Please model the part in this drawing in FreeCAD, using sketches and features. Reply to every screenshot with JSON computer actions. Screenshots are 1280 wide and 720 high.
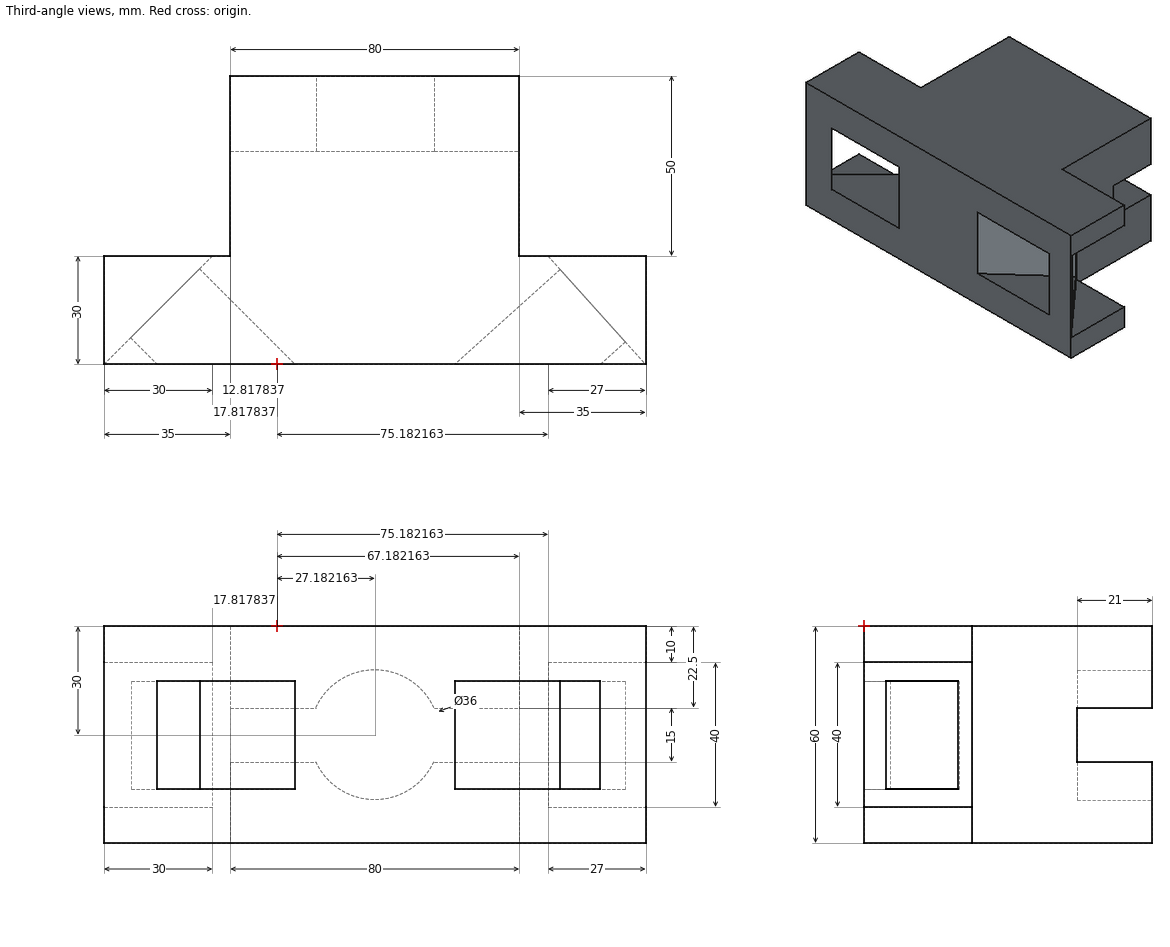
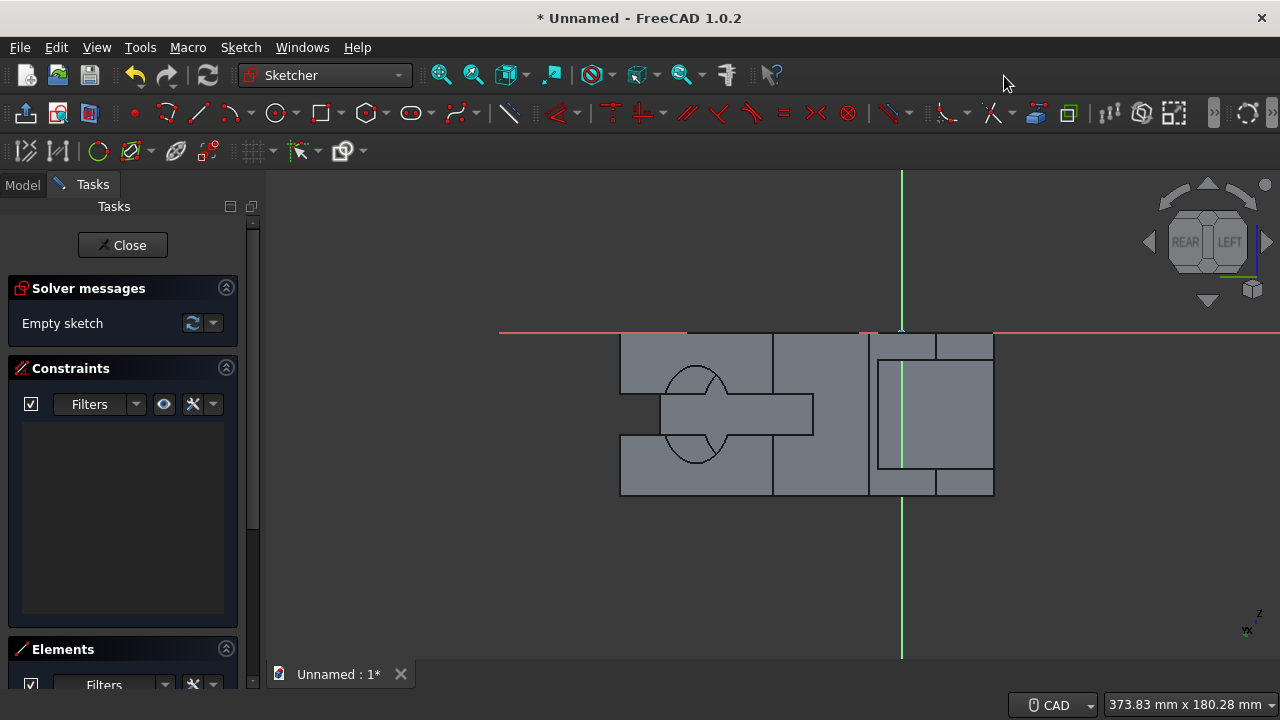
{"action": "left_click", "coordinate": [90, 114]}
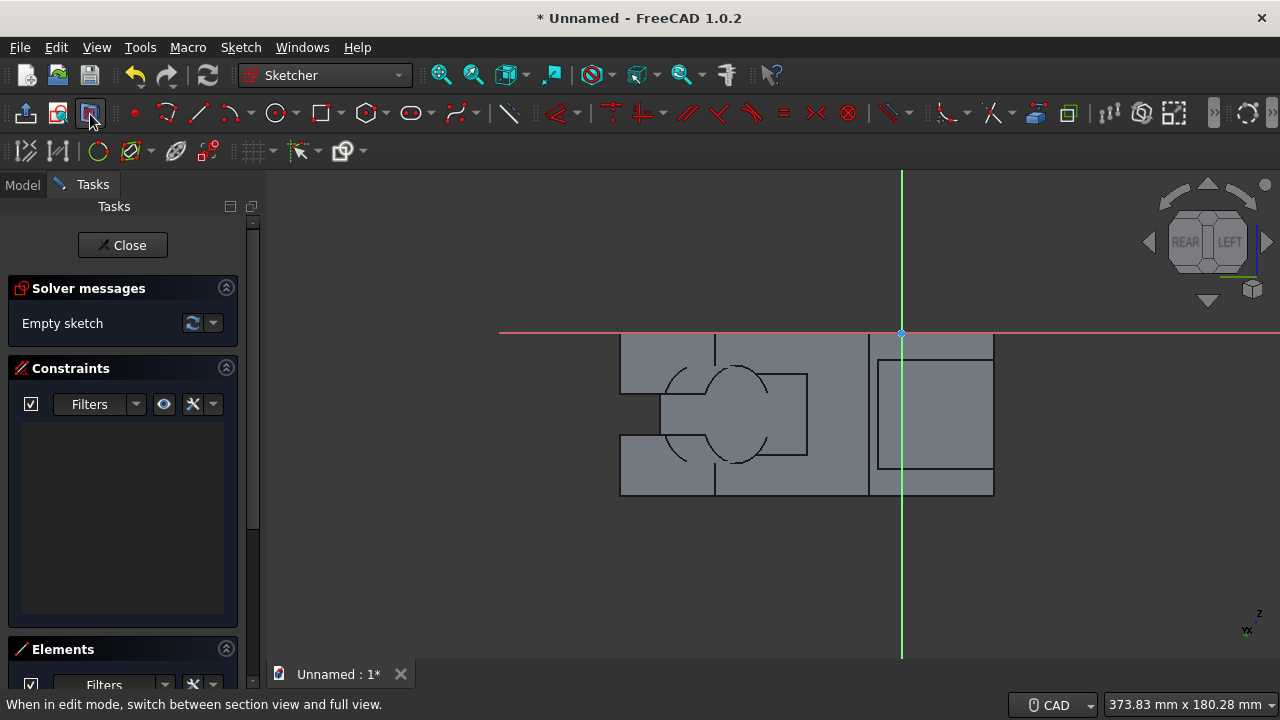
{"action": "scroll", "coordinate": [1059, 382], "scroll_direction": "up", "scroll_amount": 5}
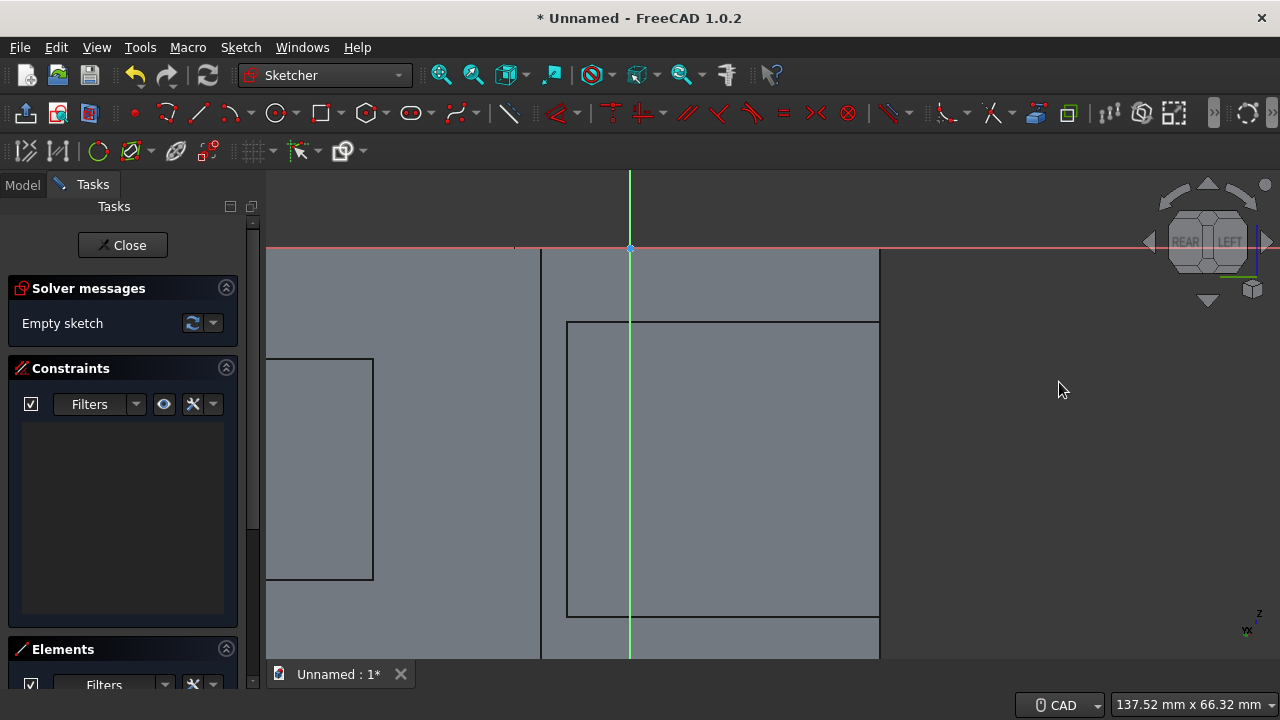
{"action": "left_click", "coordinate": [322, 114]}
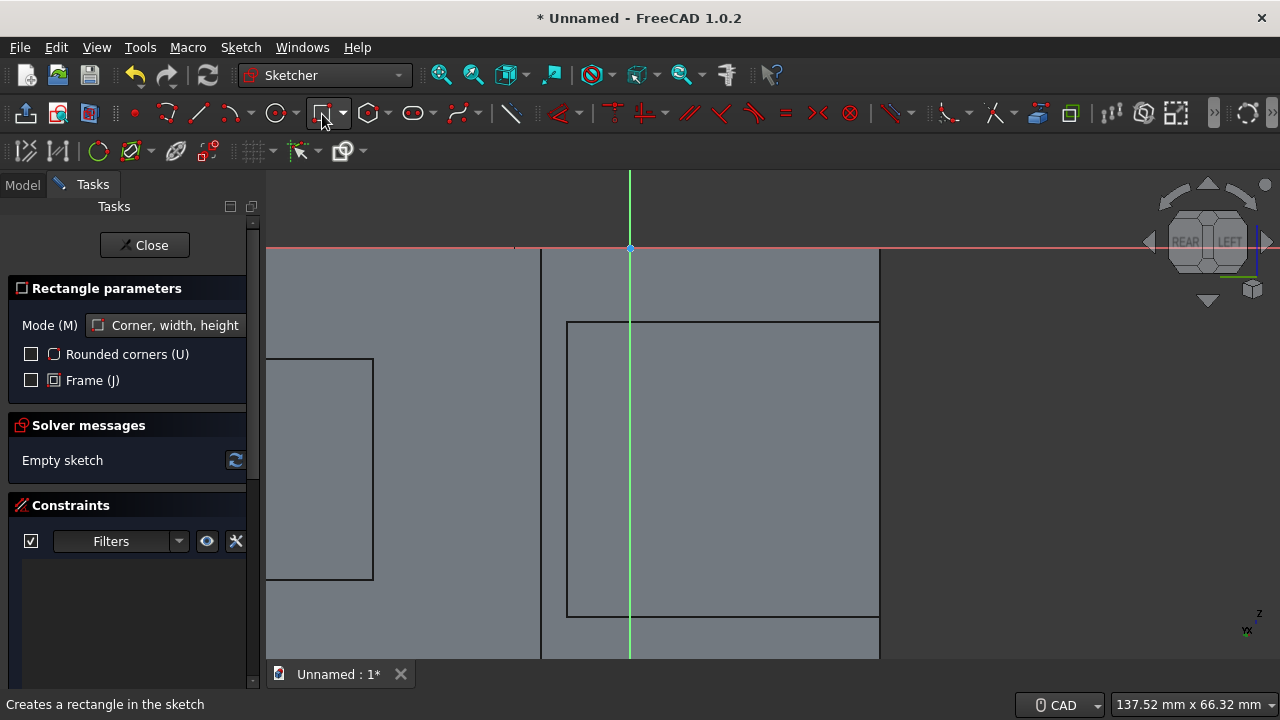
{"action": "left_click", "coordinate": [604, 359]}
{"action": "left_click", "coordinate": [803, 580]}
{"action": "key", "text": "Escape"}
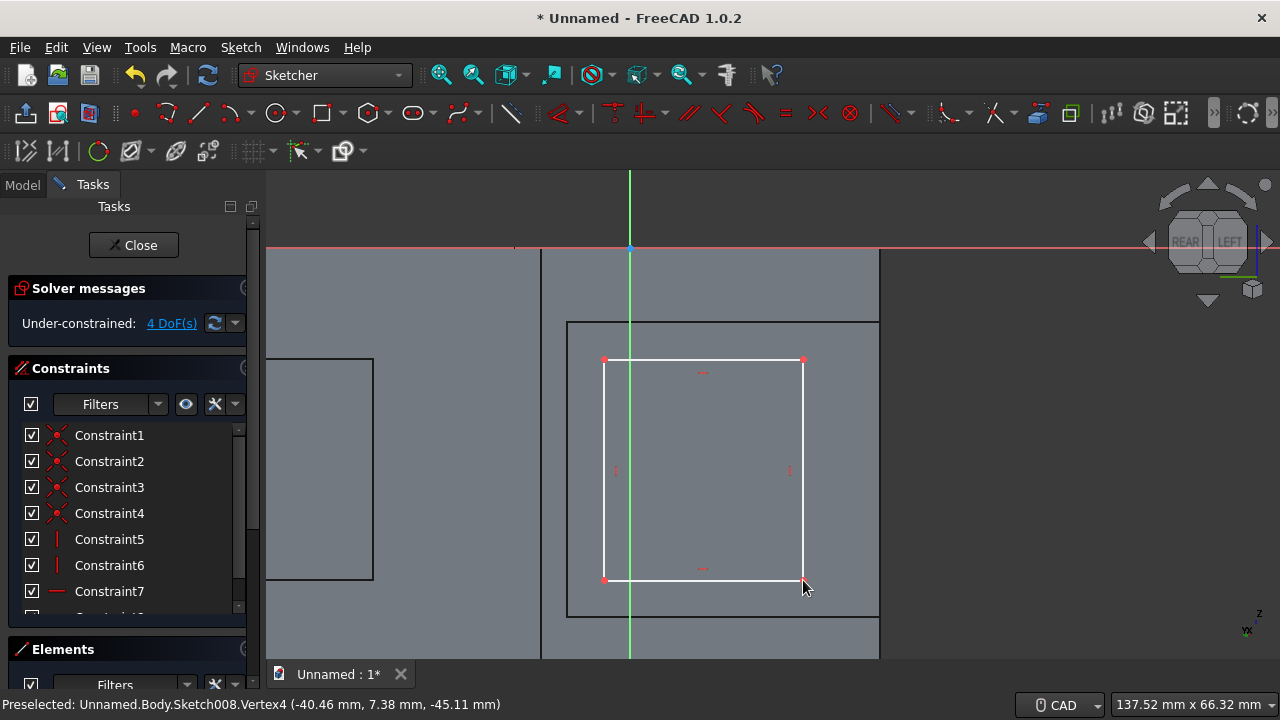
{"action": "left_click", "coordinate": [558, 114]}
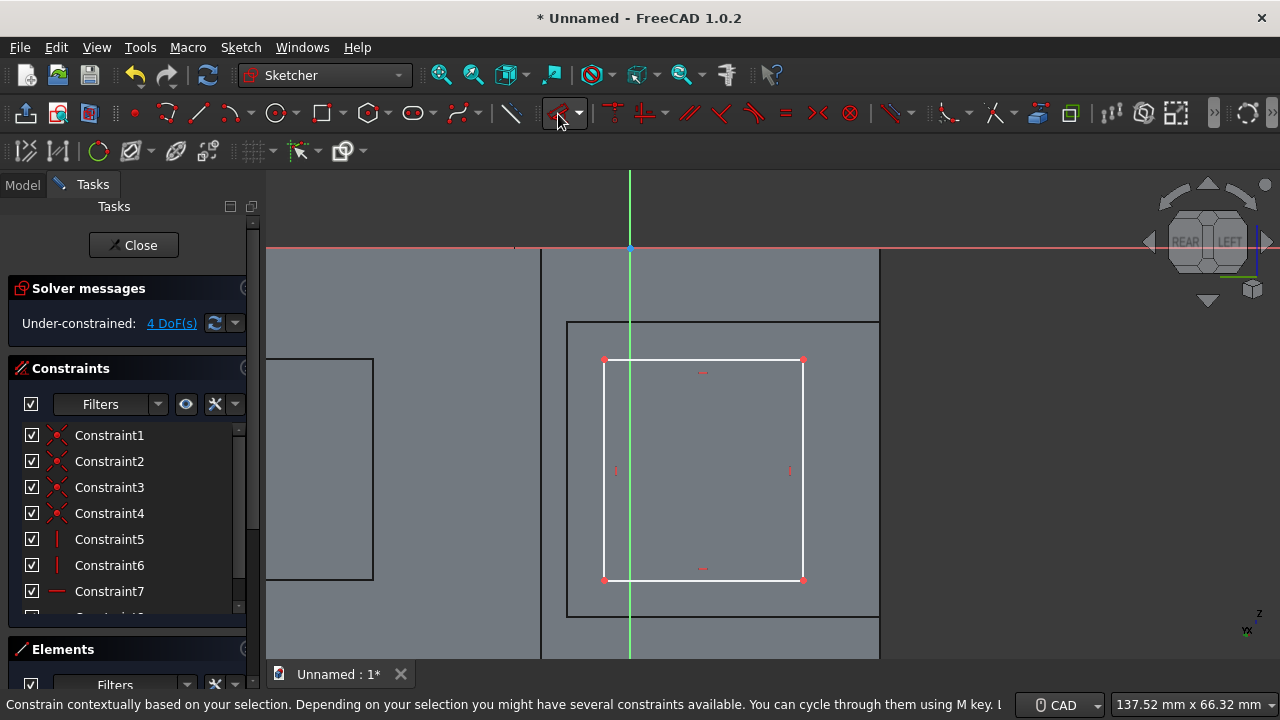
{"action": "left_click", "coordinate": [604, 426]}
{"action": "left_click", "coordinate": [570, 471]}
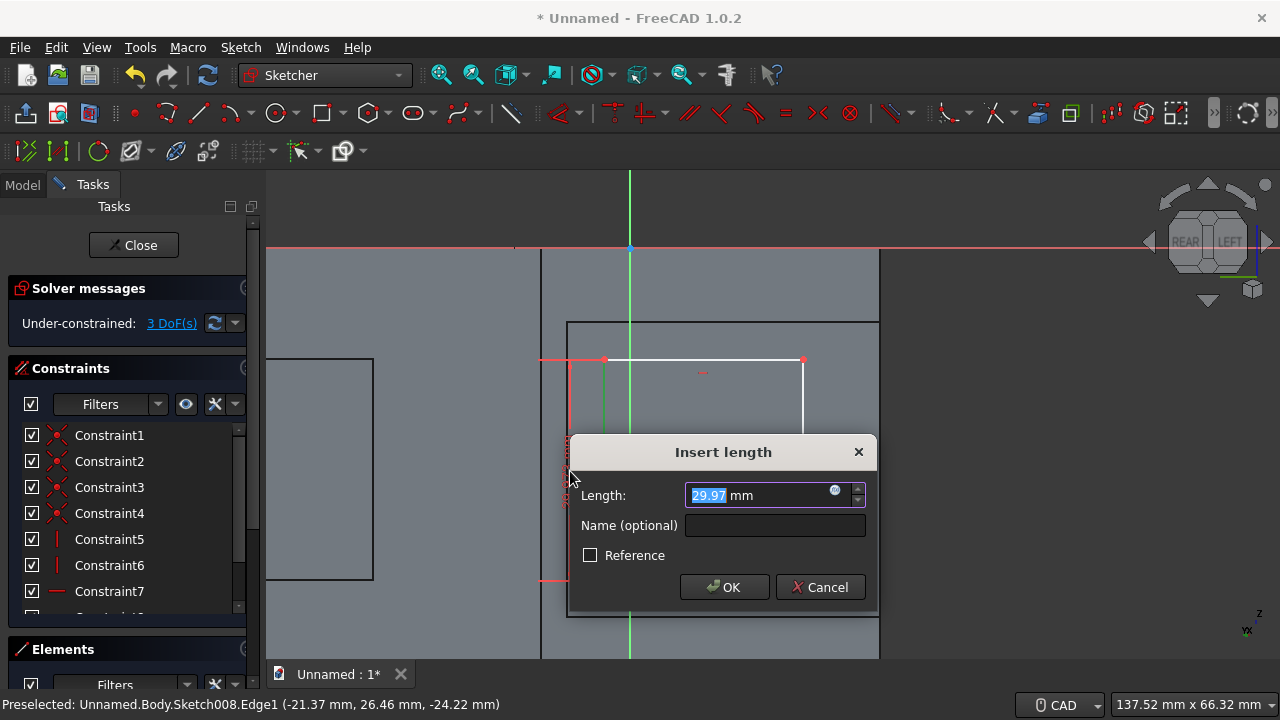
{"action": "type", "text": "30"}
{"action": "key", "text": "Return"}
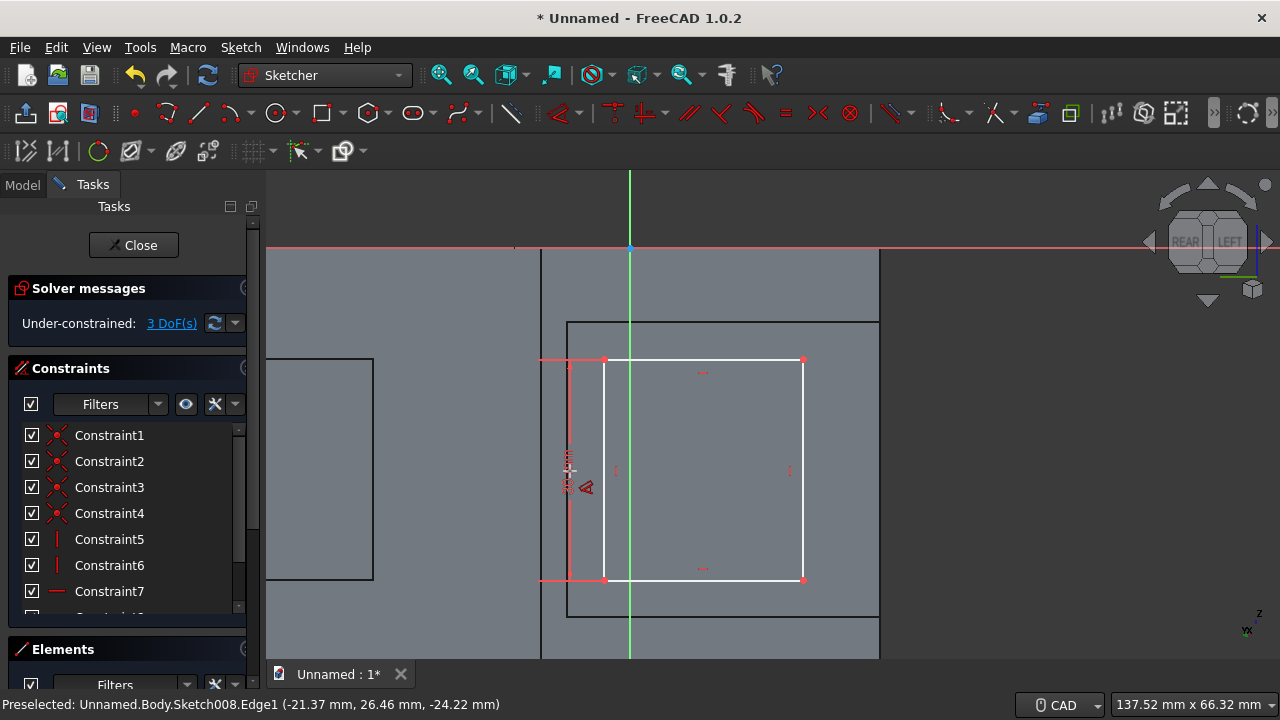
{"action": "left_click", "coordinate": [664, 581]}
{"action": "left_click", "coordinate": [703, 615]}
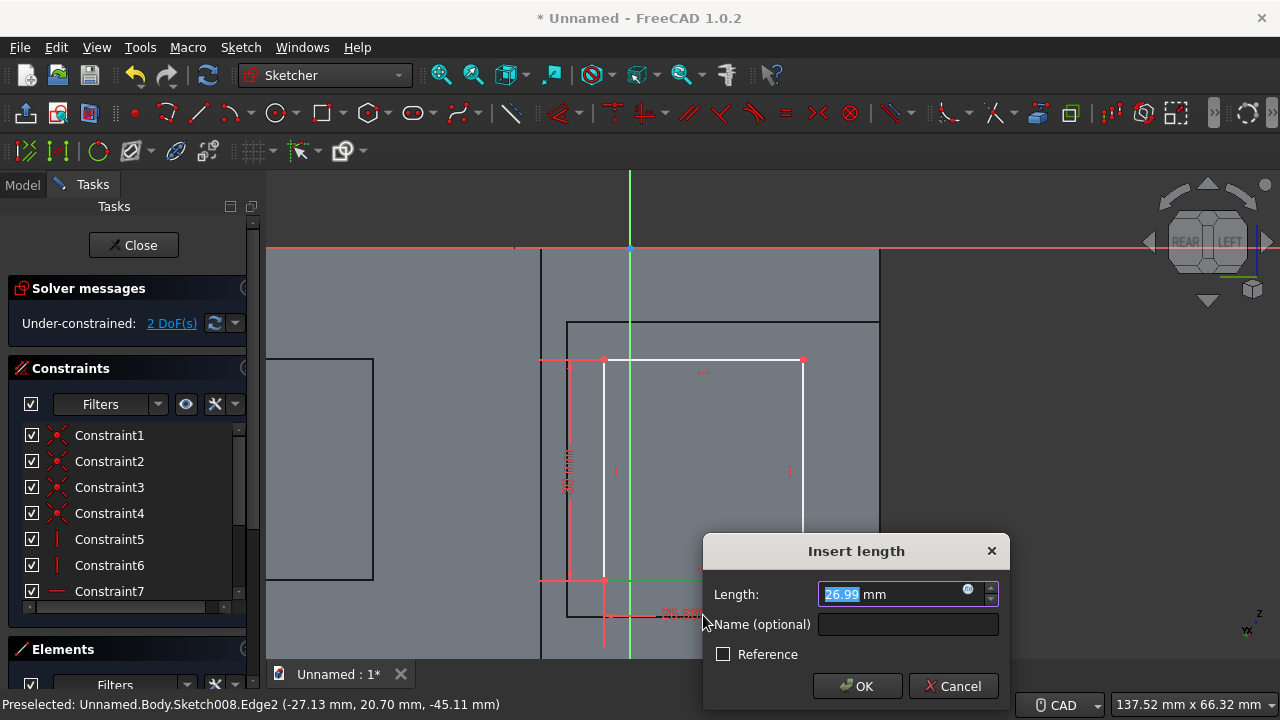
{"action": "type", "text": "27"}
{"action": "key", "text": "Return"}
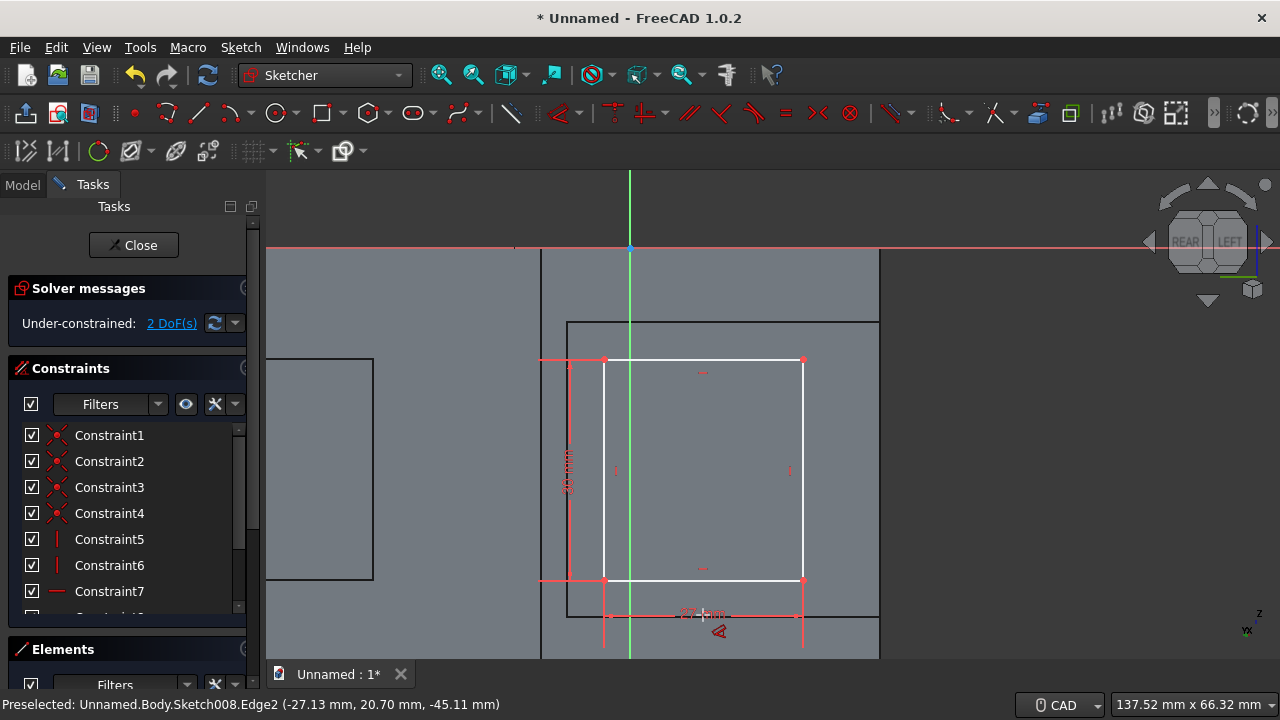
{"action": "left_click", "coordinate": [604, 360]}
{"action": "left_click", "coordinate": [570, 304]}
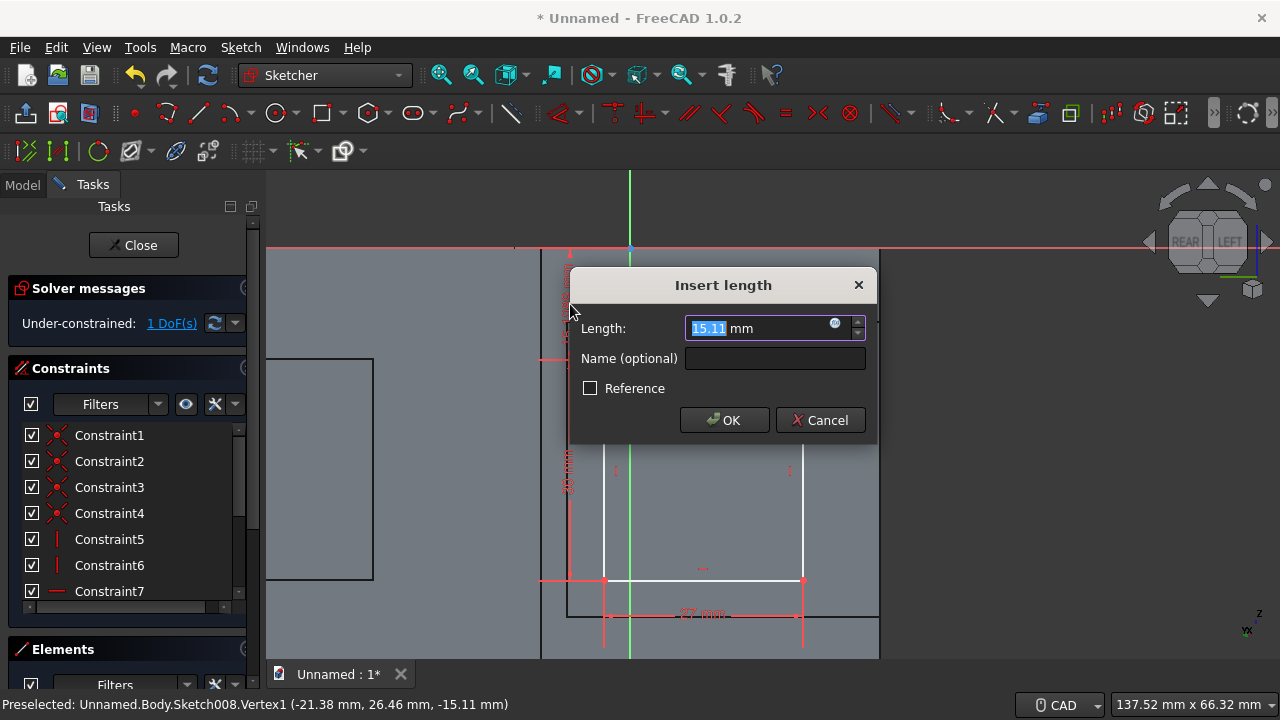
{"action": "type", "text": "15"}
{"action": "key", "text": "Return"}